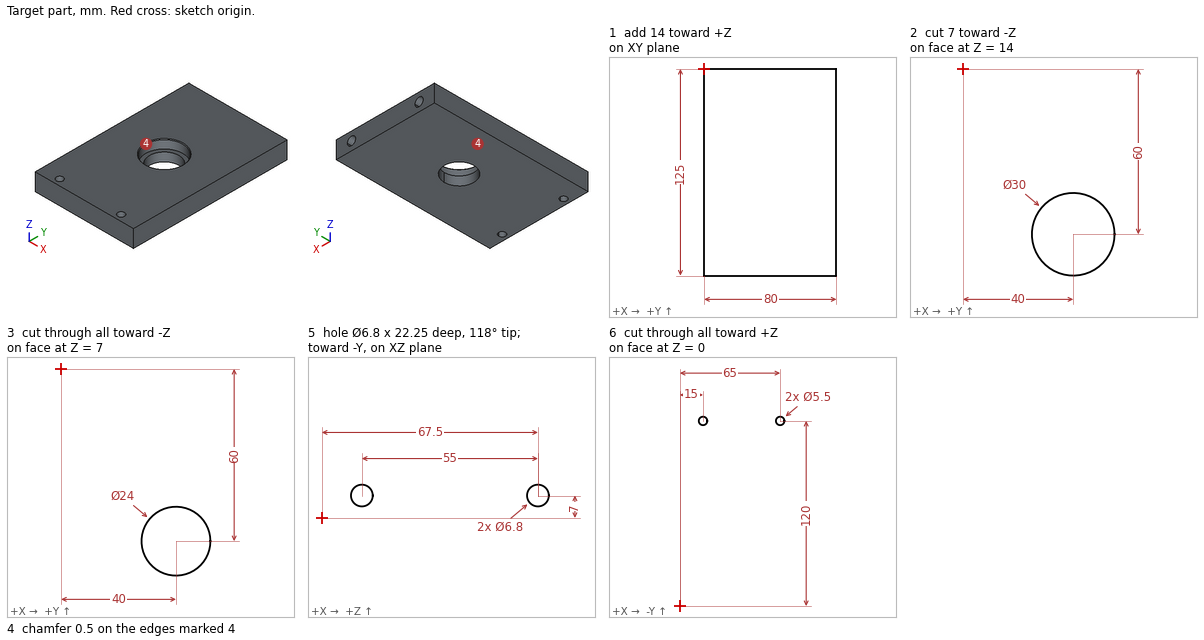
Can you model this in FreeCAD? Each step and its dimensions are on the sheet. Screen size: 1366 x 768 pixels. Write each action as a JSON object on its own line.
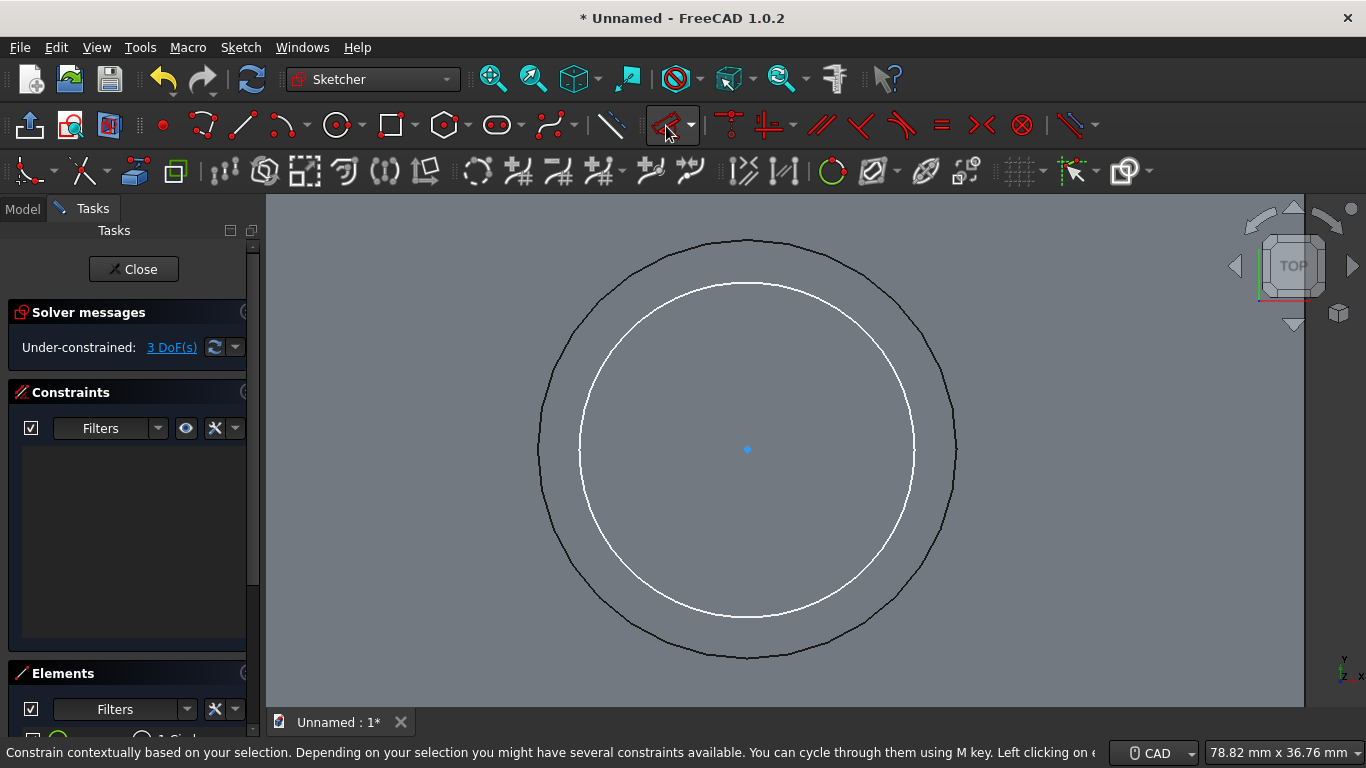
{"action": "left_click", "coordinate": [865, 331]}
{"action": "left_click", "coordinate": [888, 308]}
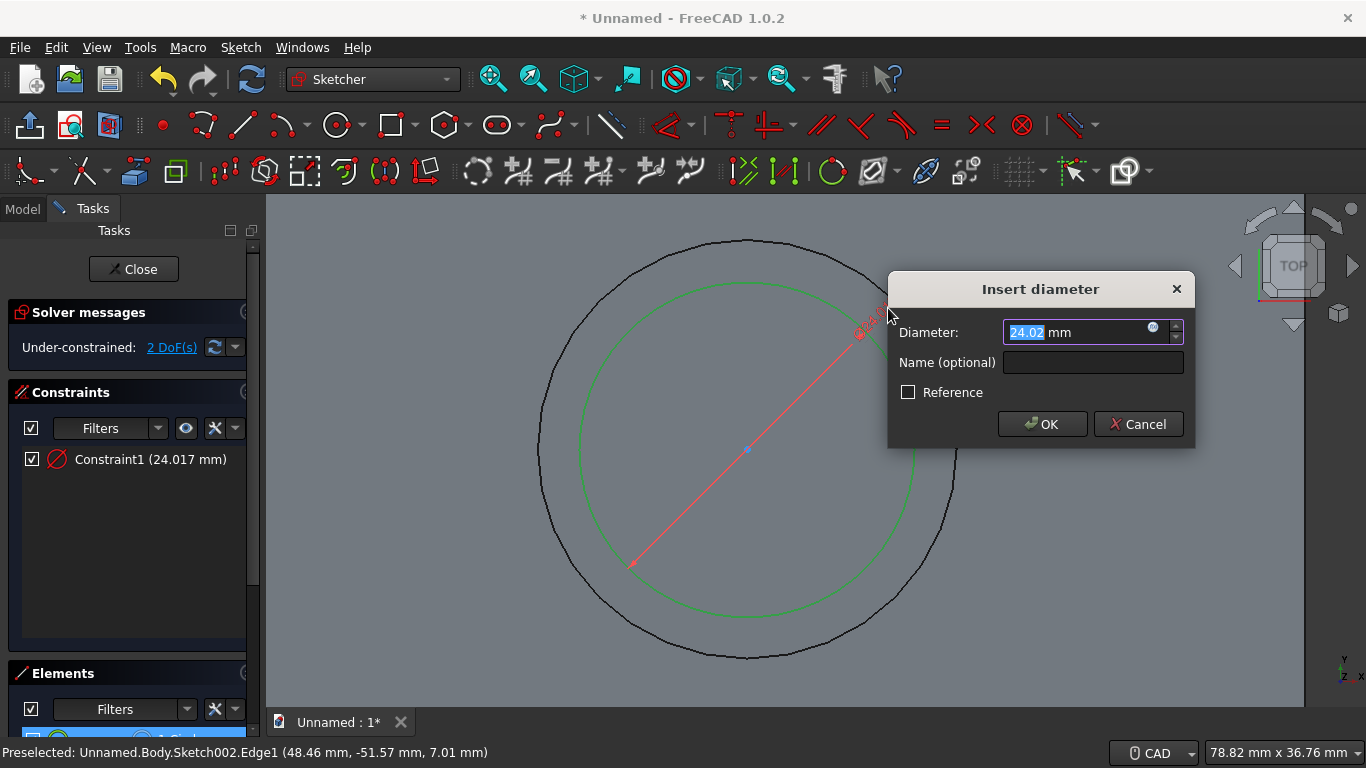
{"action": "type", "text": "24"}
{"action": "key", "text": "Return"}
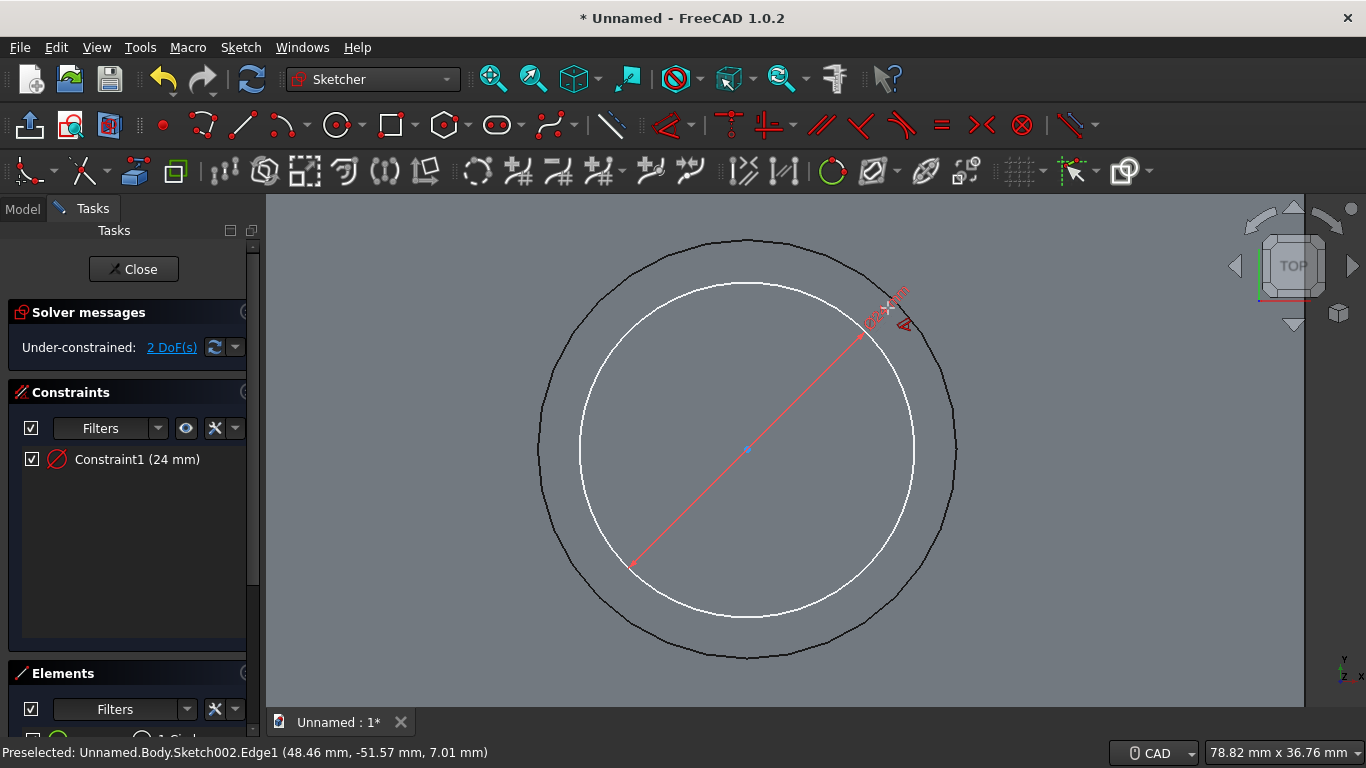
{"action": "left_click", "coordinate": [747, 450]}
{"action": "left_click", "coordinate": [520, 484]}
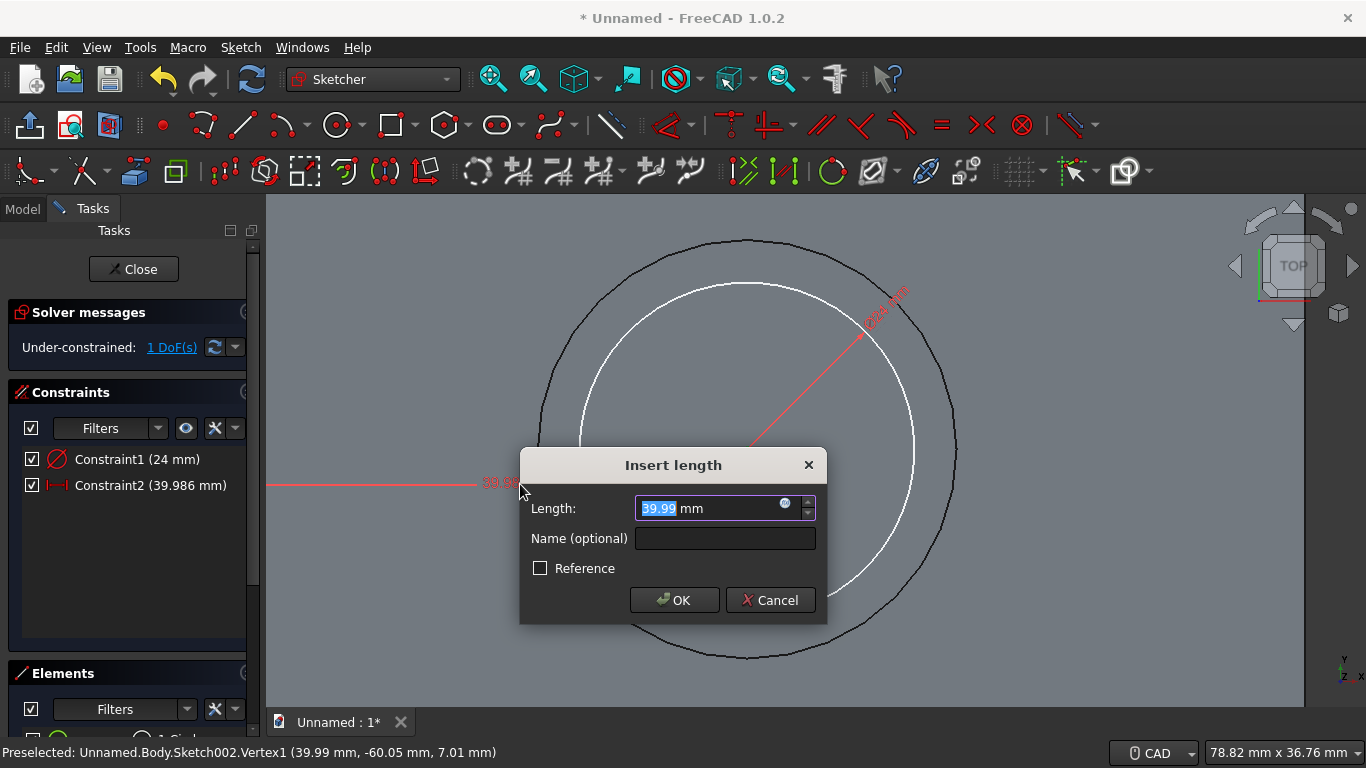
{"action": "type", "text": "40"}
{"action": "key", "text": "Return"}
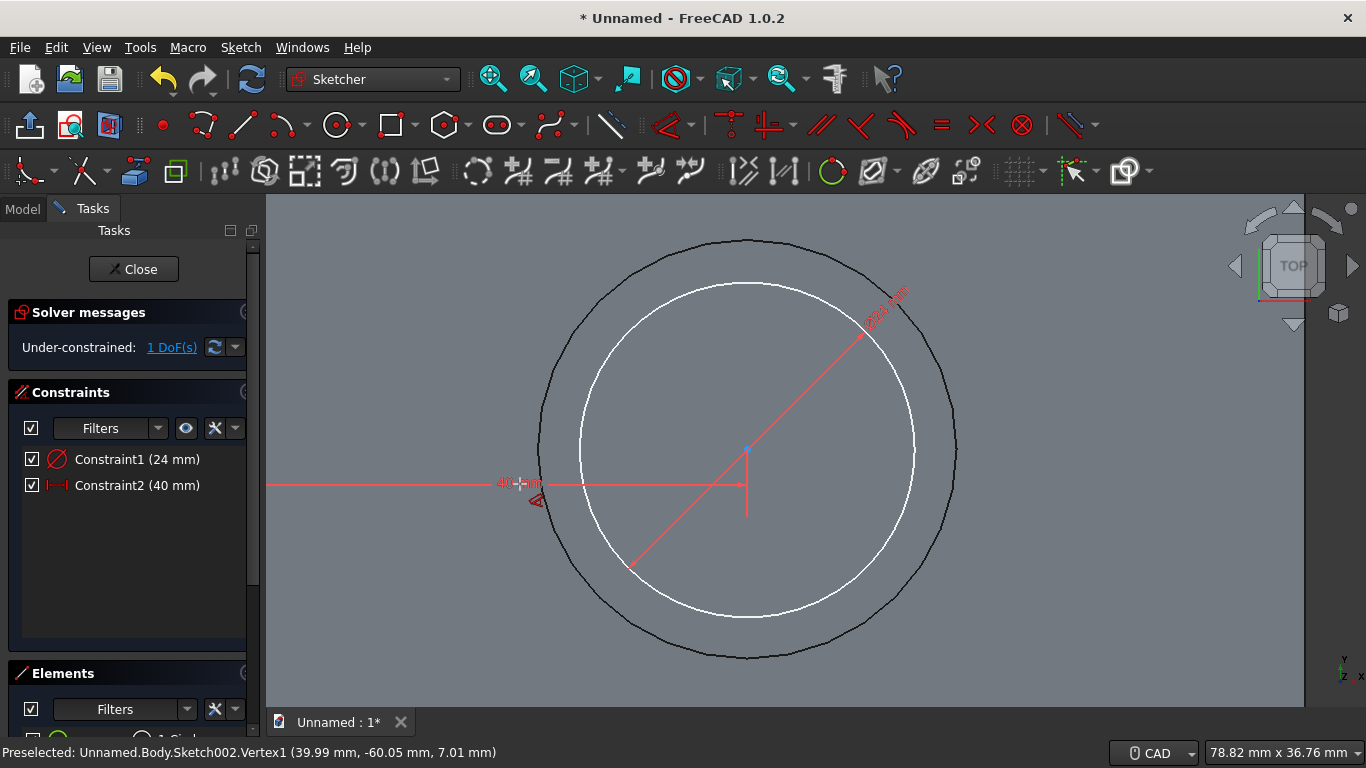
{"action": "left_click", "coordinate": [747, 450]}
{"action": "left_click", "coordinate": [781, 336]}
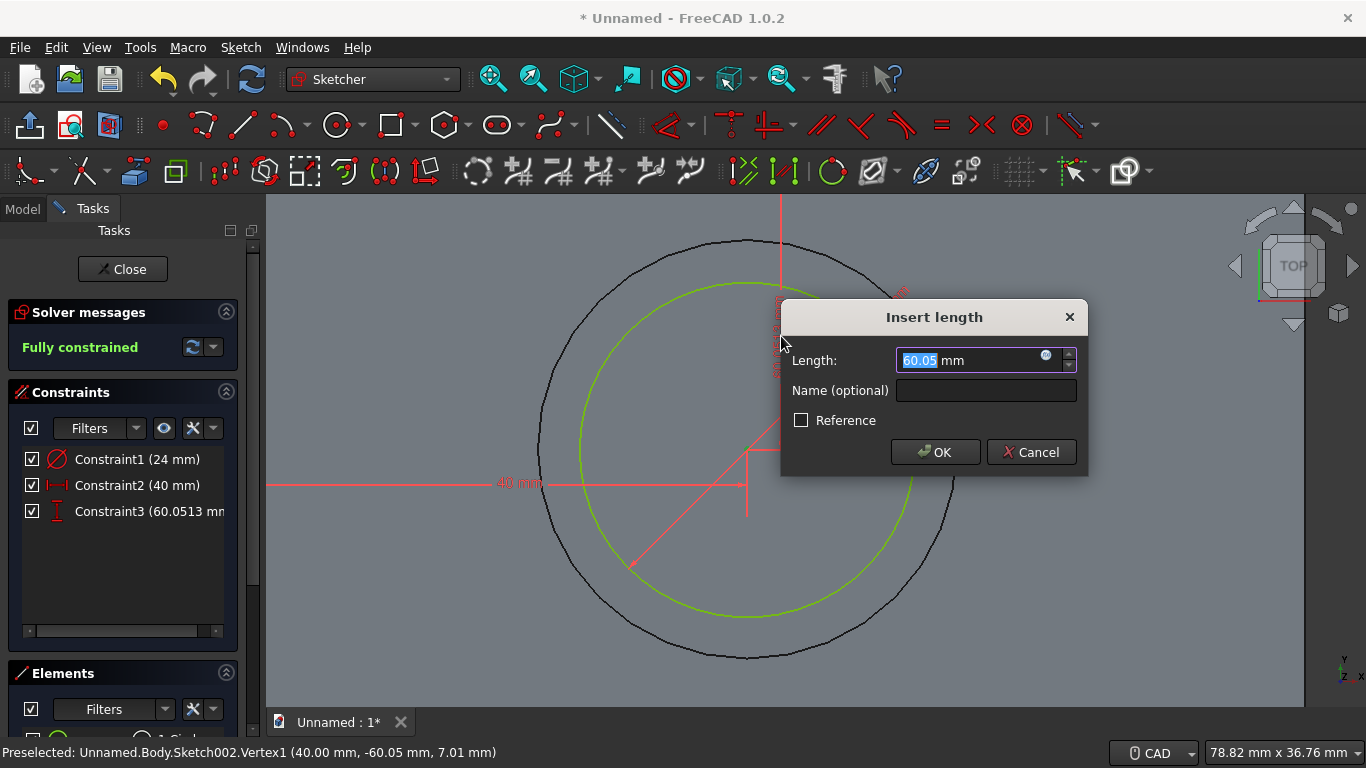
{"action": "type", "text": "60"}
{"action": "key", "text": "Return"}
{"action": "key", "text": "Escape"}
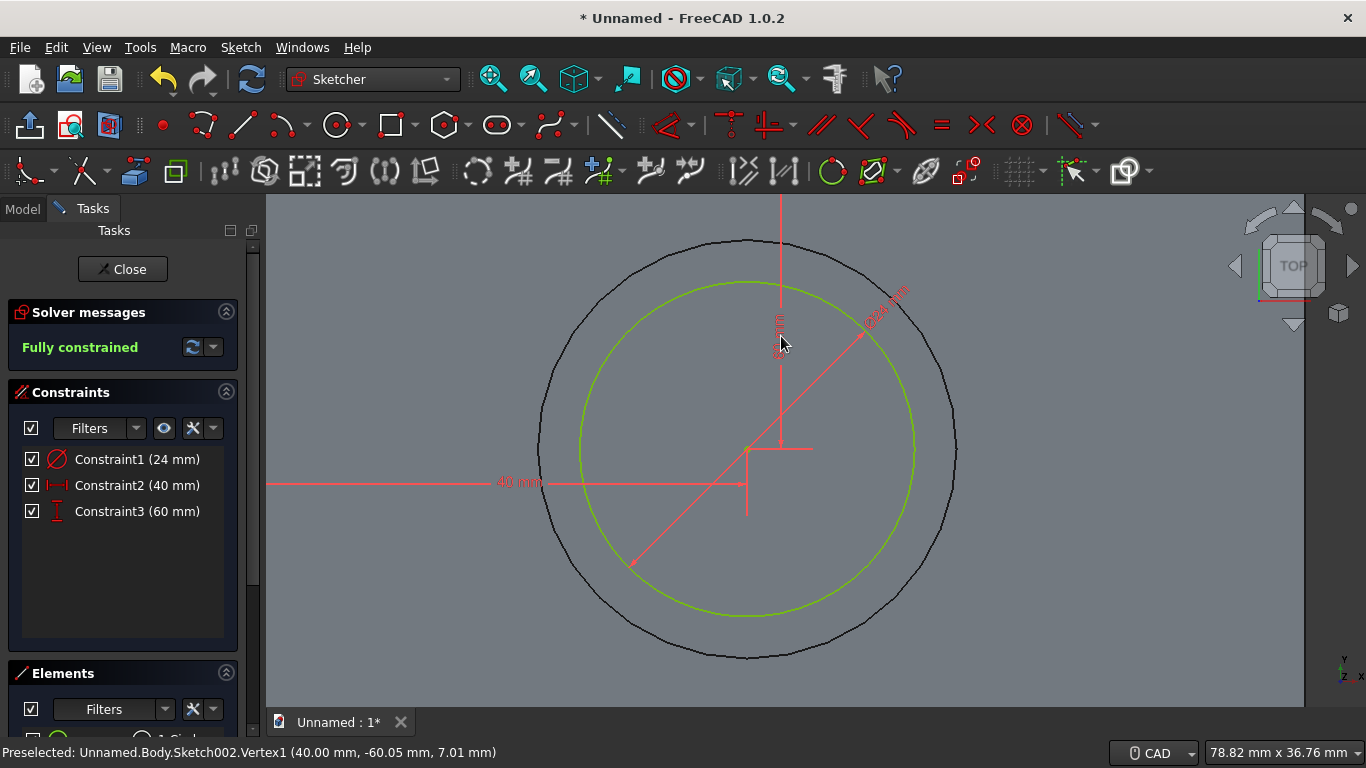
{"action": "left_click", "coordinate": [123, 269]}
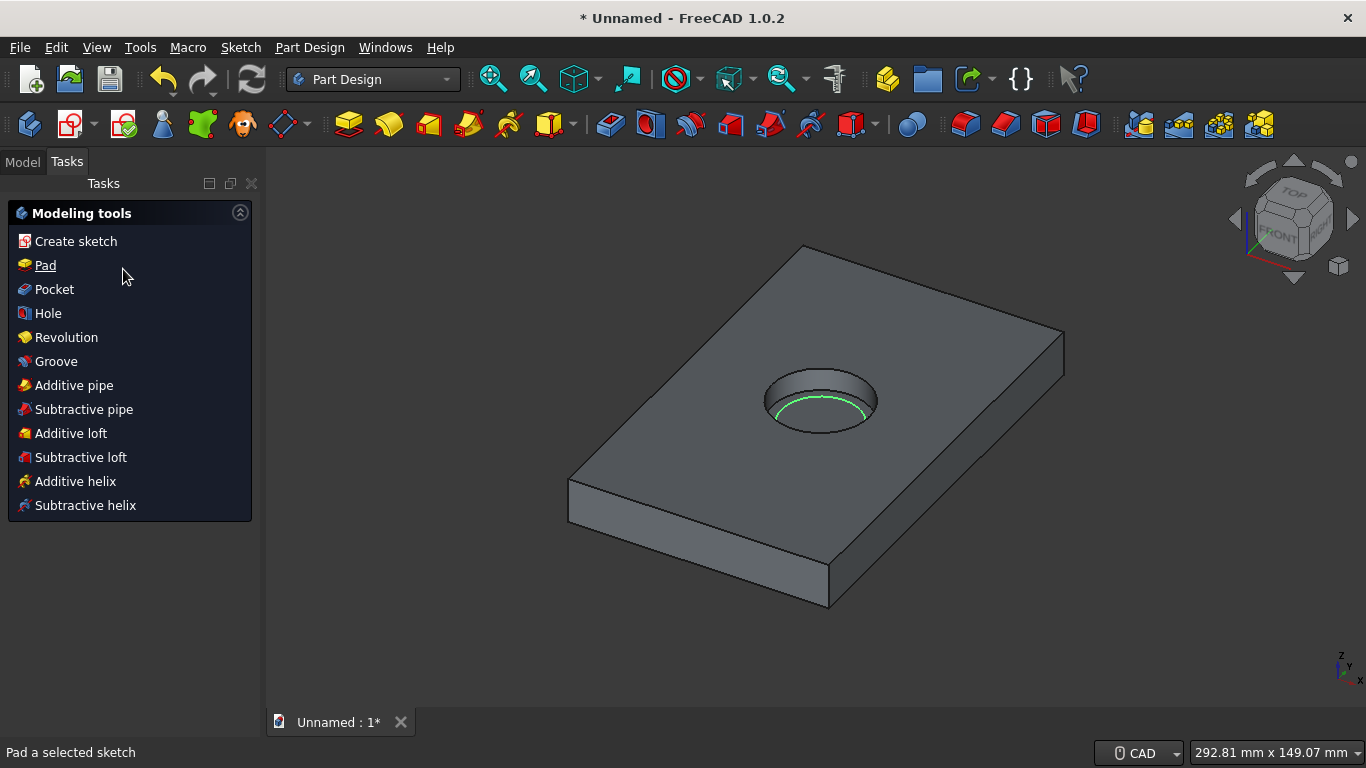
{"action": "left_click", "coordinate": [612, 124]}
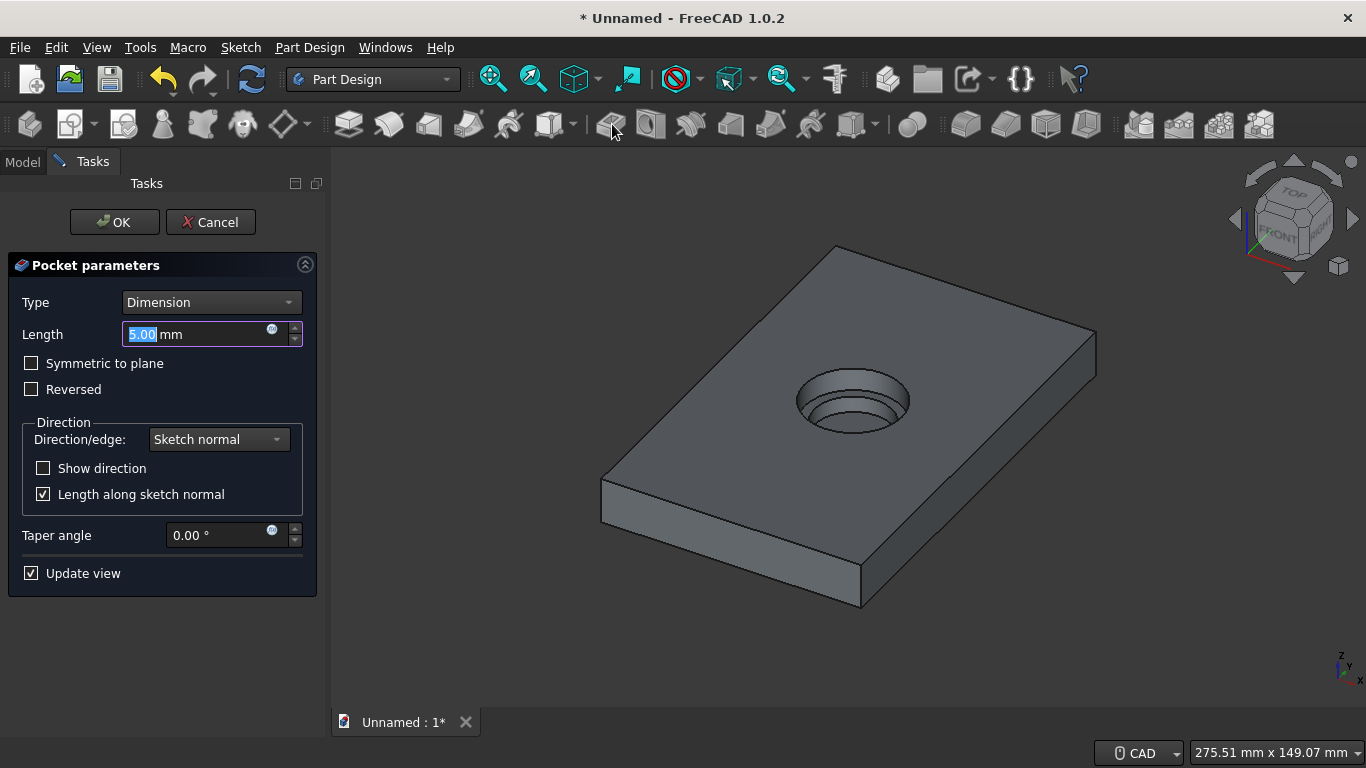
{"action": "left_click", "coordinate": [212, 302]}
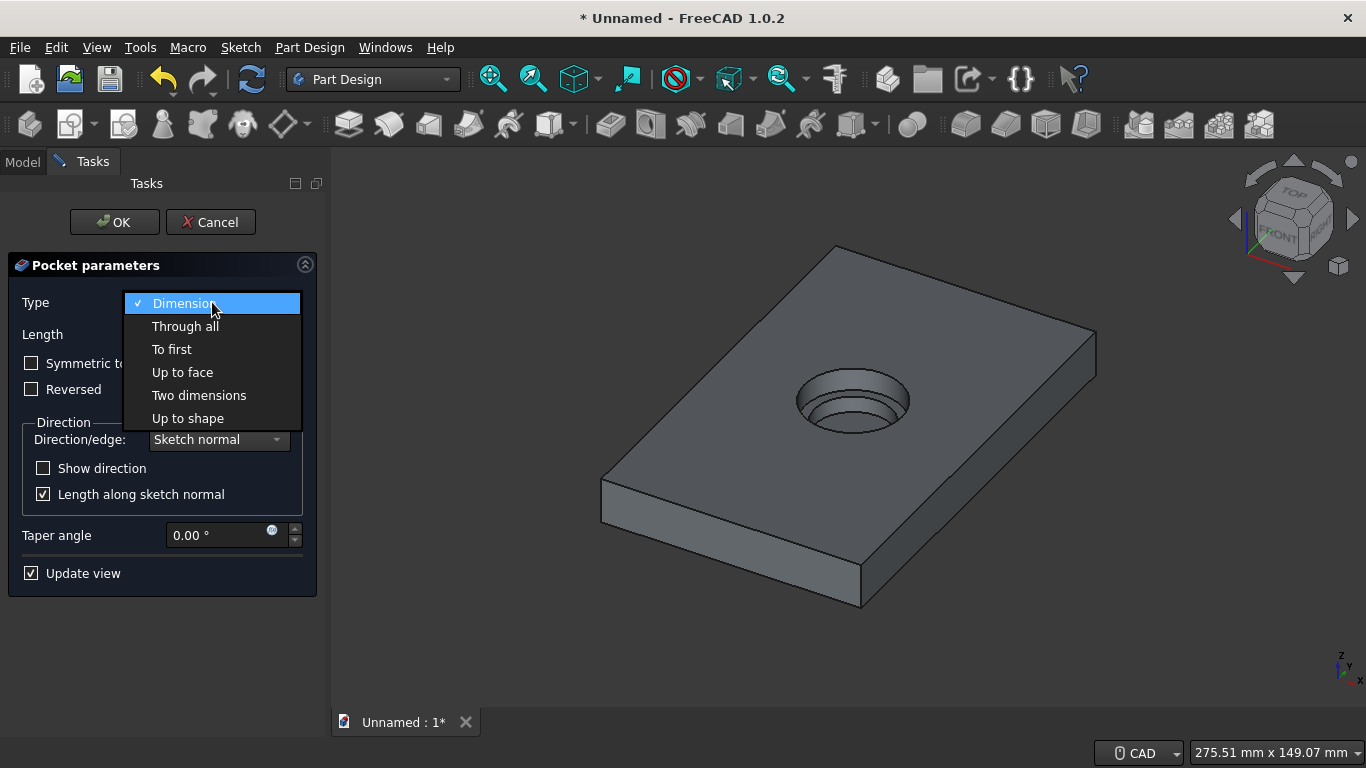
{"action": "left_click", "coordinate": [212, 326]}